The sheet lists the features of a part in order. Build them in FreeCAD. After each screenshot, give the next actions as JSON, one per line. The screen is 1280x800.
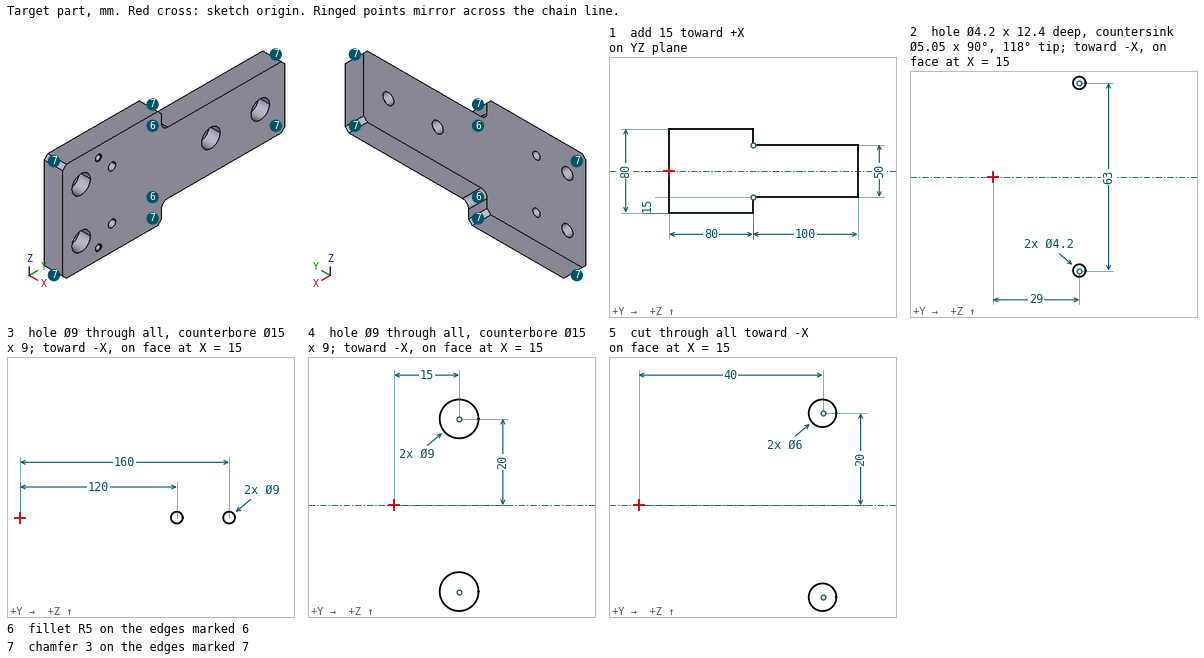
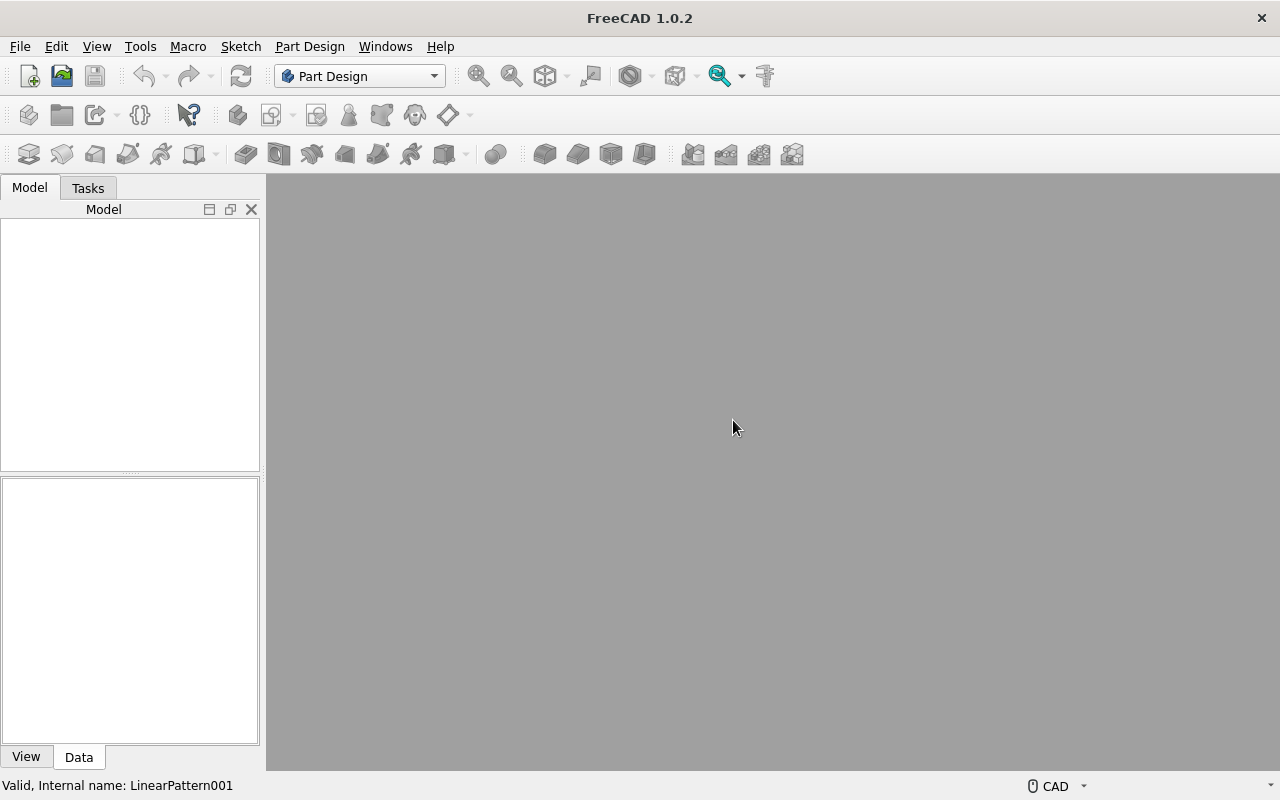
{"action": "left_click", "coordinate": [29, 76]}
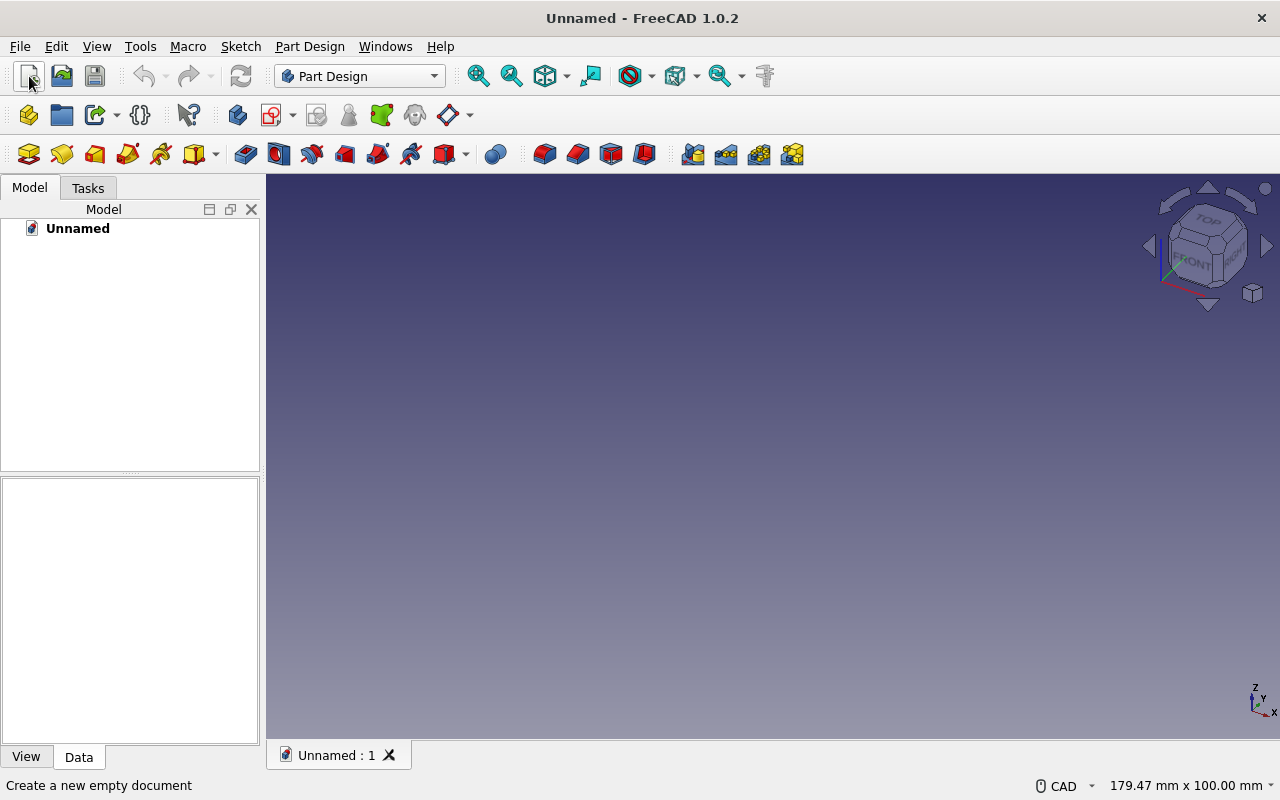
{"action": "left_click", "coordinate": [270, 116]}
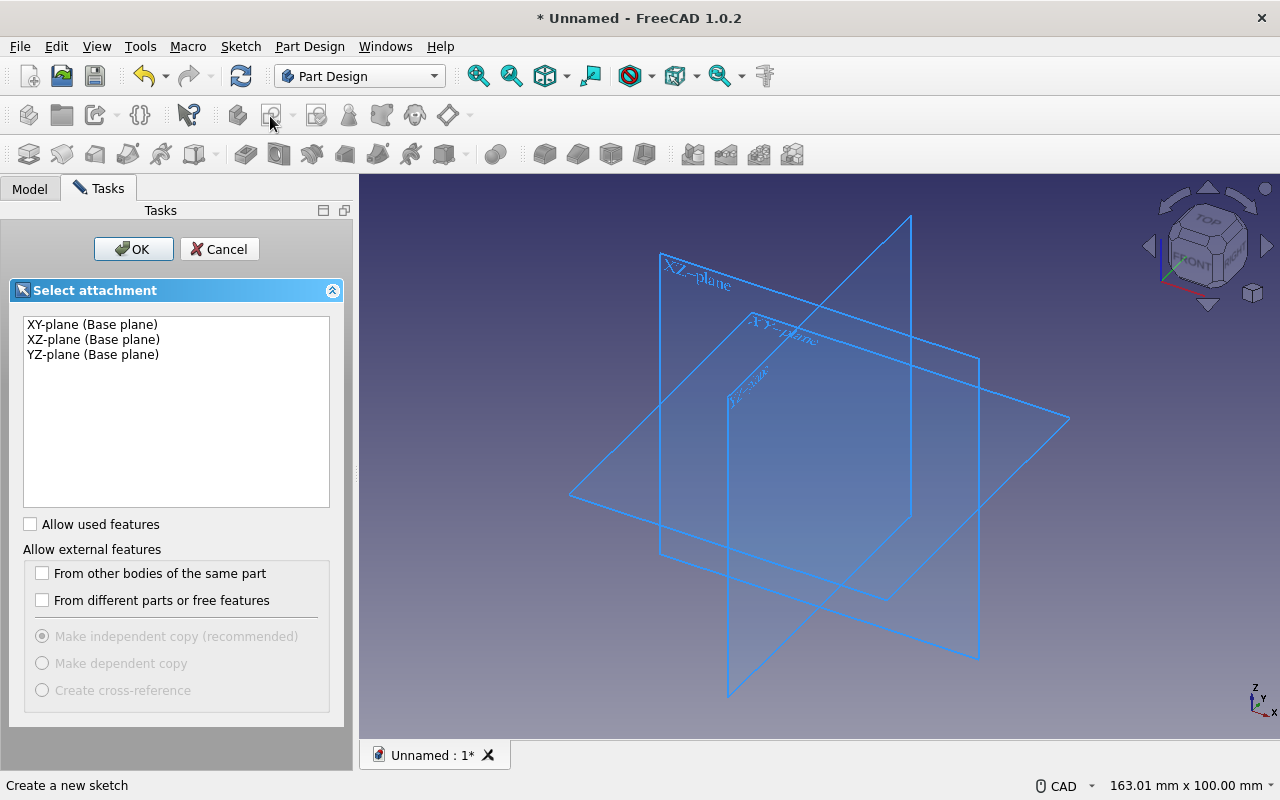
{"action": "left_click", "coordinate": [84, 354]}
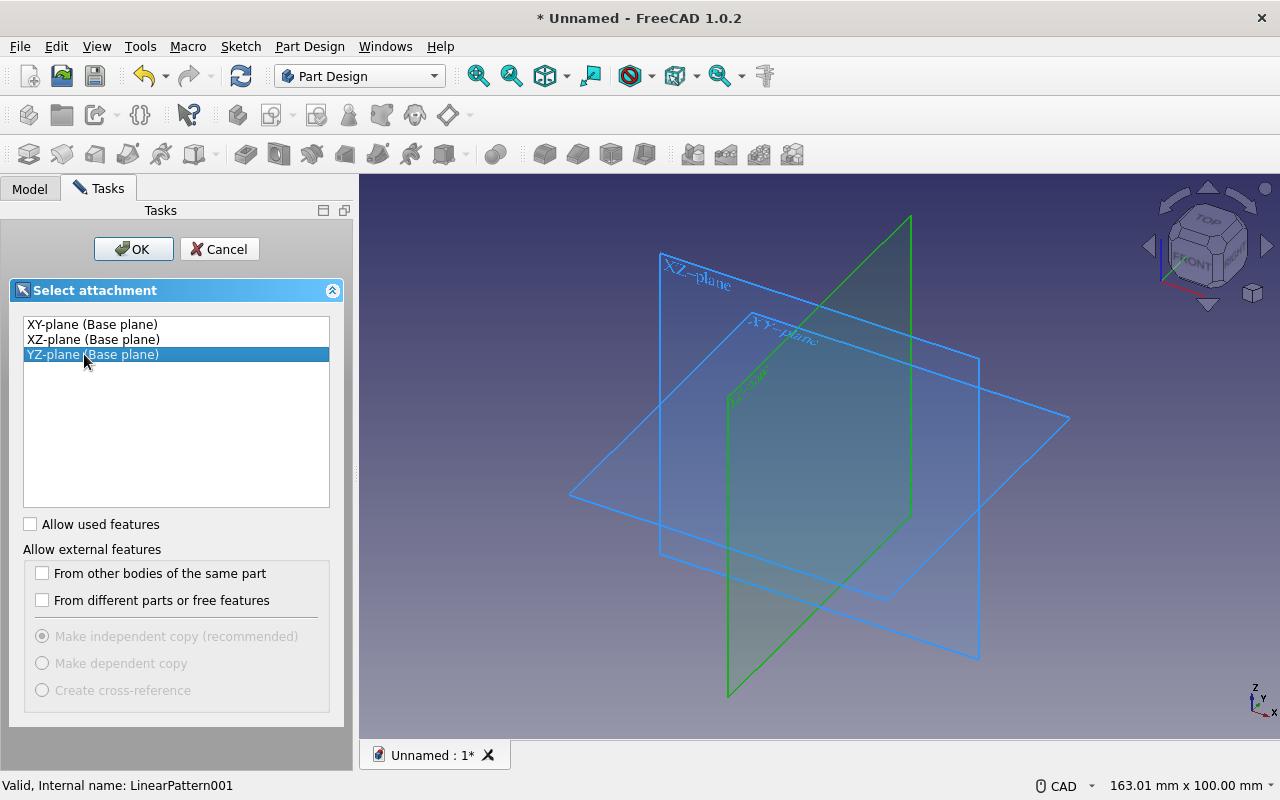
{"action": "left_click", "coordinate": [134, 249]}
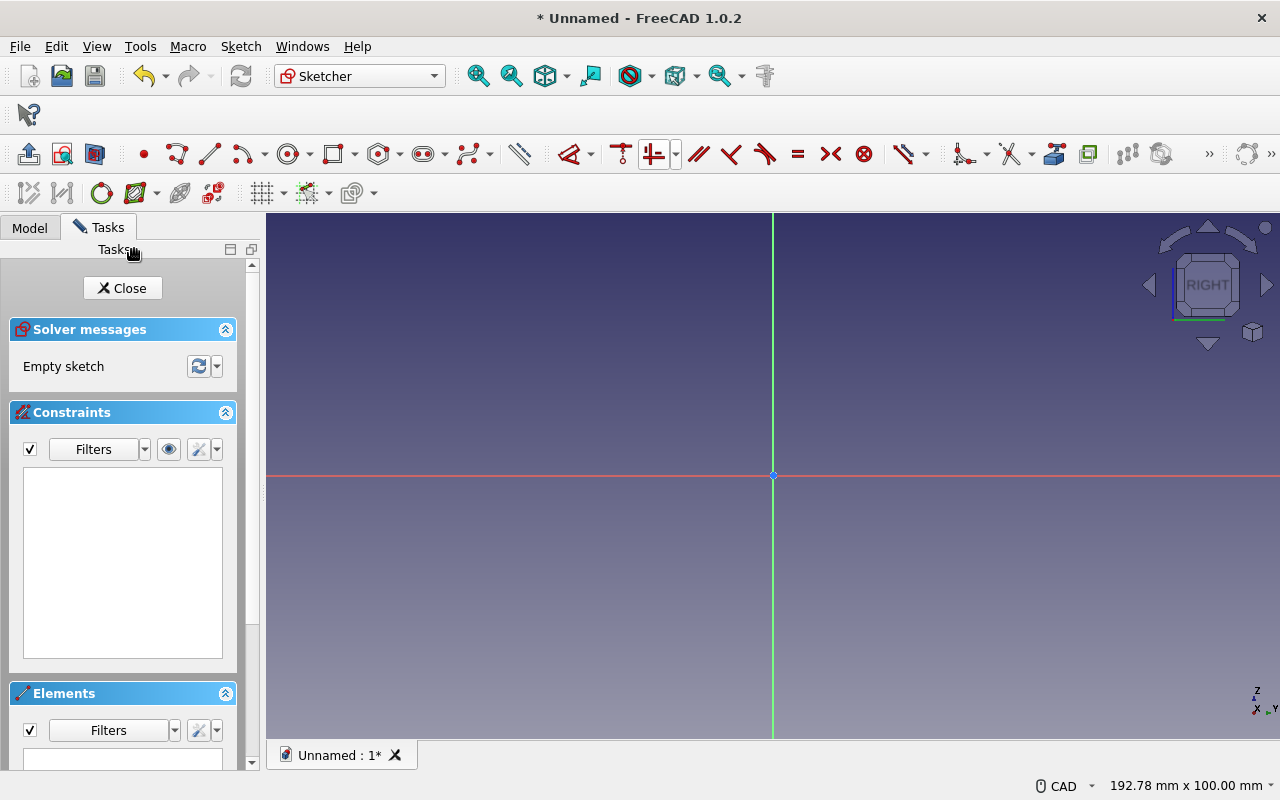
{"action": "scroll", "coordinate": [294, 476], "scroll_direction": "down", "scroll_amount": 3}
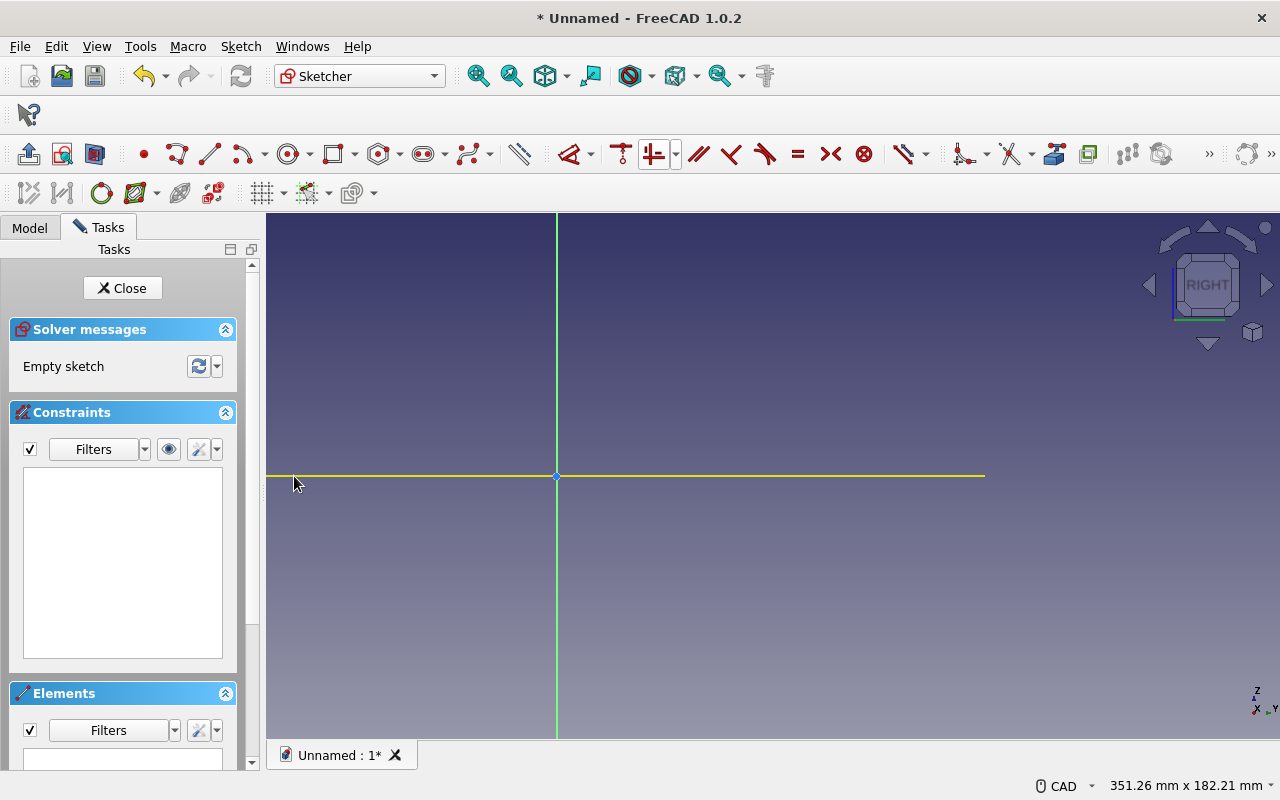
{"action": "left_click", "coordinate": [177, 154]}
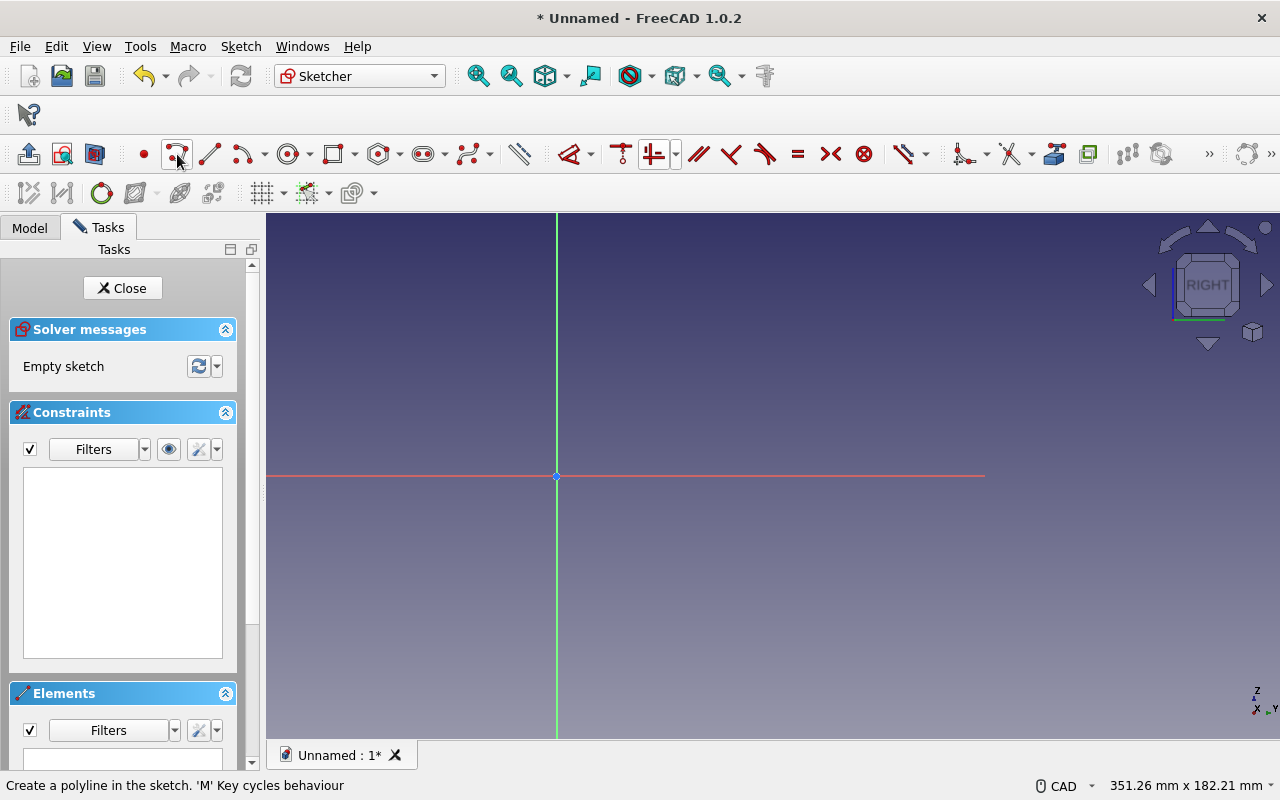
{"action": "left_click", "coordinate": [557, 361]}
{"action": "left_click", "coordinate": [566, 592]}
{"action": "left_click", "coordinate": [788, 592]}
{"action": "left_click", "coordinate": [788, 548]}
{"action": "left_click", "coordinate": [1077, 548]}
{"action": "left_click", "coordinate": [1077, 404]}
{"action": "left_click", "coordinate": [788, 404]}
{"action": "left_click", "coordinate": [788, 361]}
{"action": "left_click", "coordinate": [557, 362]}
{"action": "key", "text": "Escape"}
{"action": "key", "text": "Escape"}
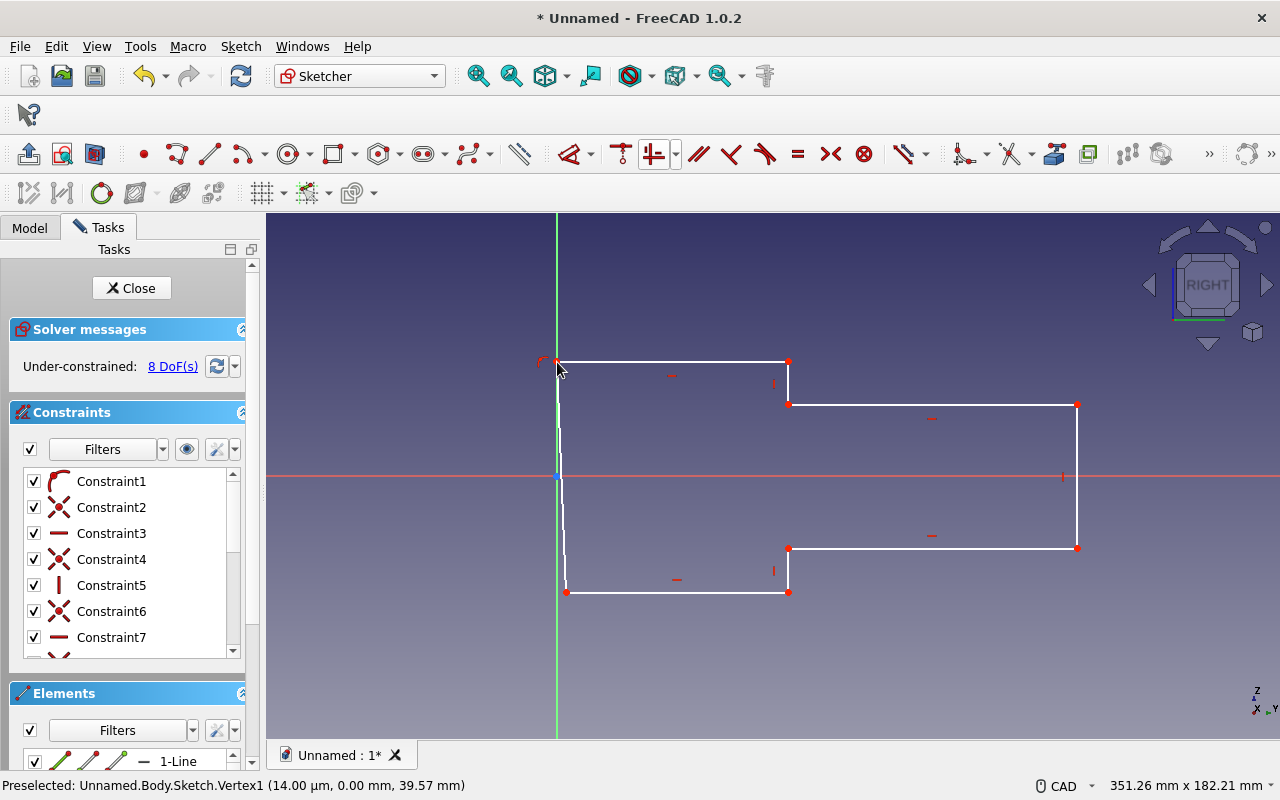
{"action": "left_click", "coordinate": [560, 431]}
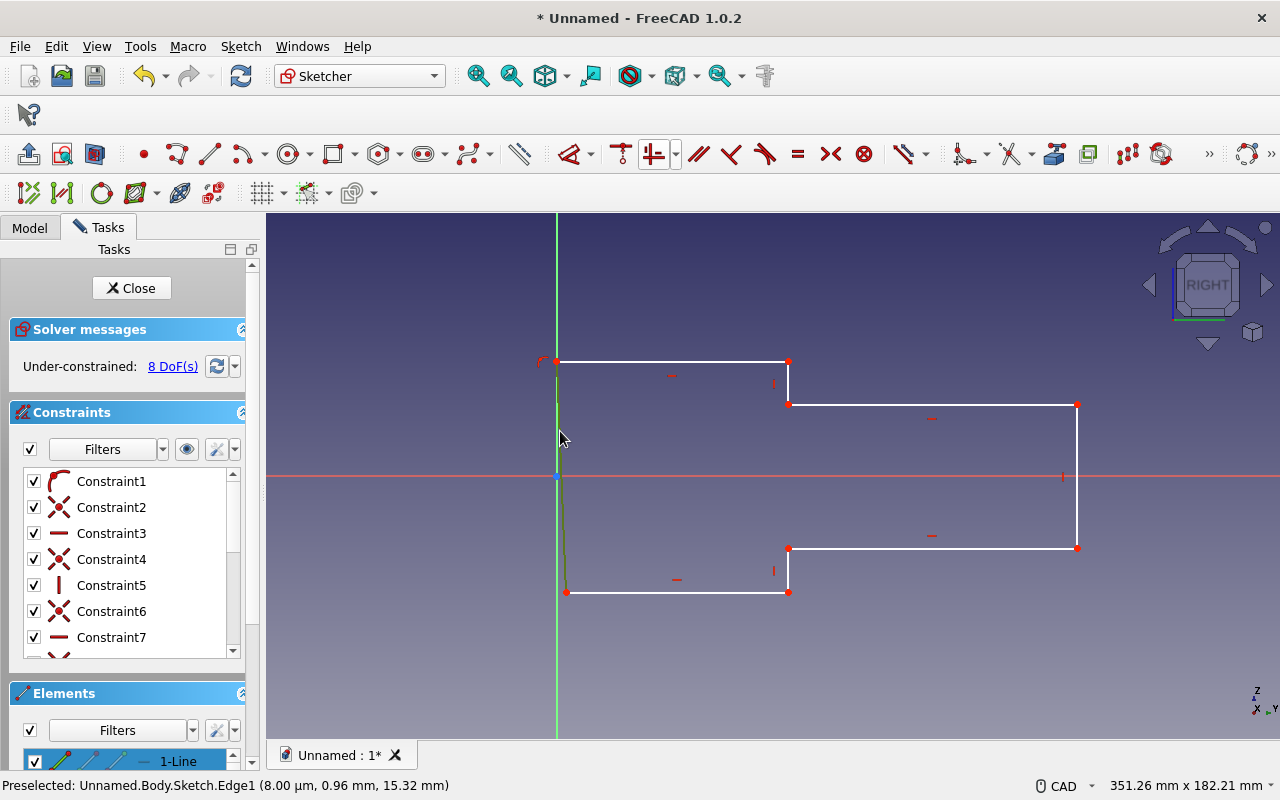
{"action": "left_click", "coordinate": [676, 154]}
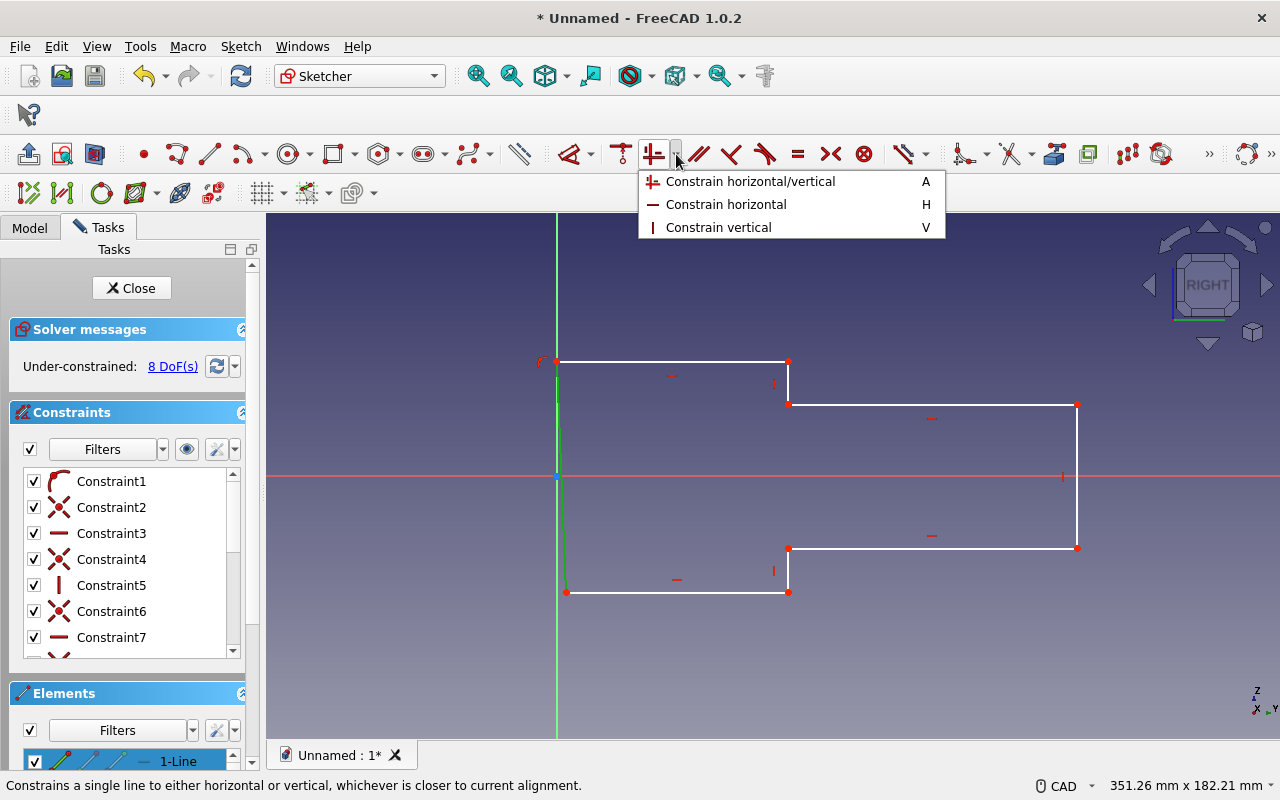
{"action": "left_click", "coordinate": [792, 228]}